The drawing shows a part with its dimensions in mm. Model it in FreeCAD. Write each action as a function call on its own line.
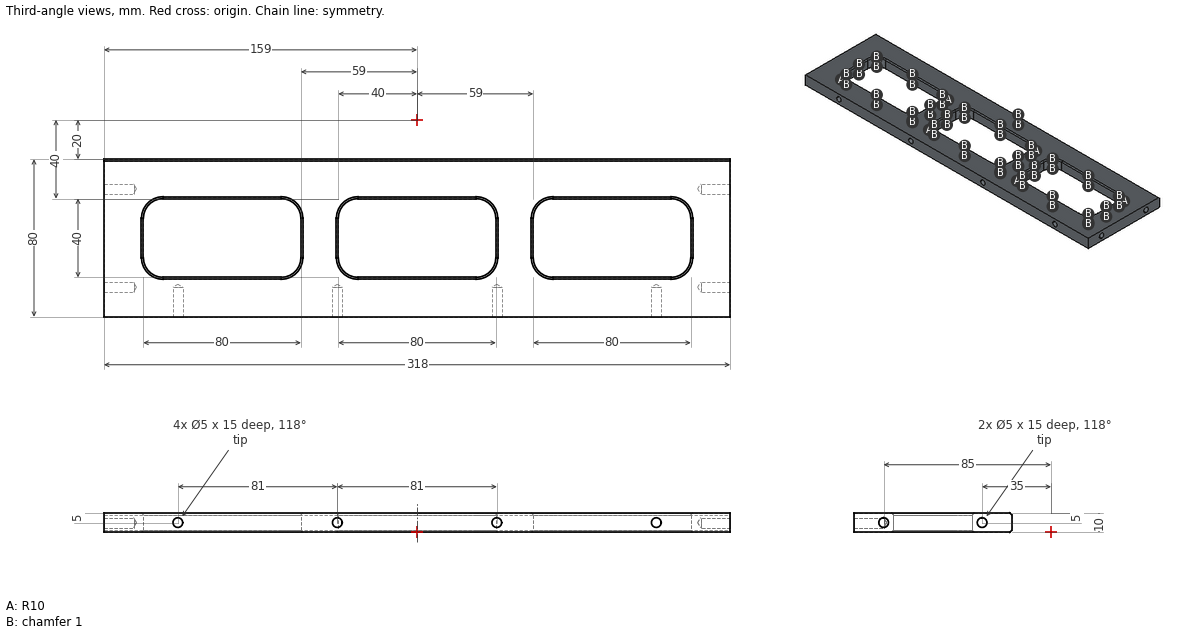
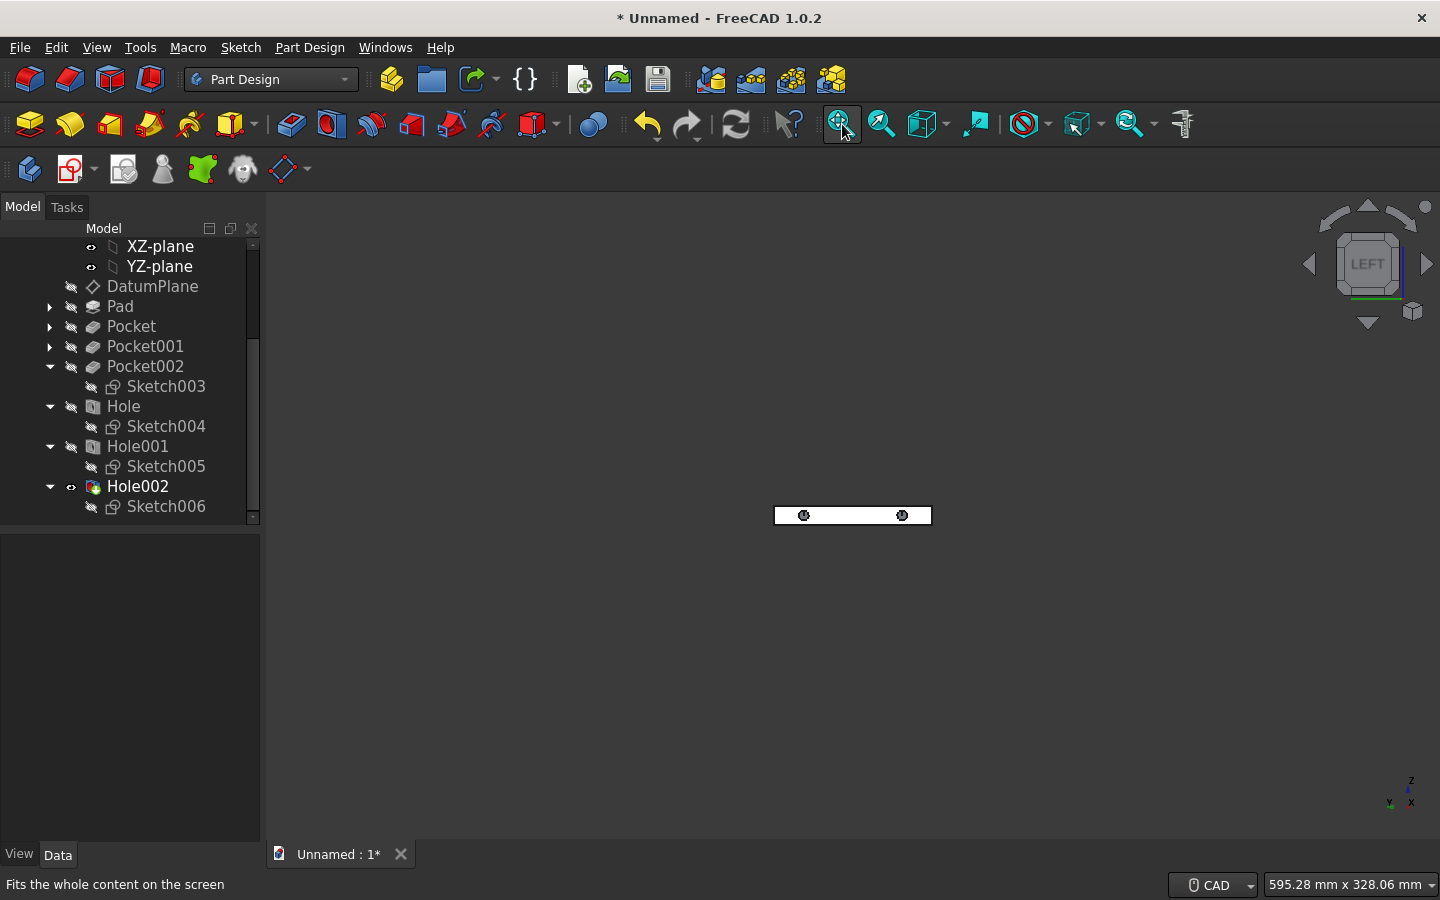
scroll(892, 514, up, 4)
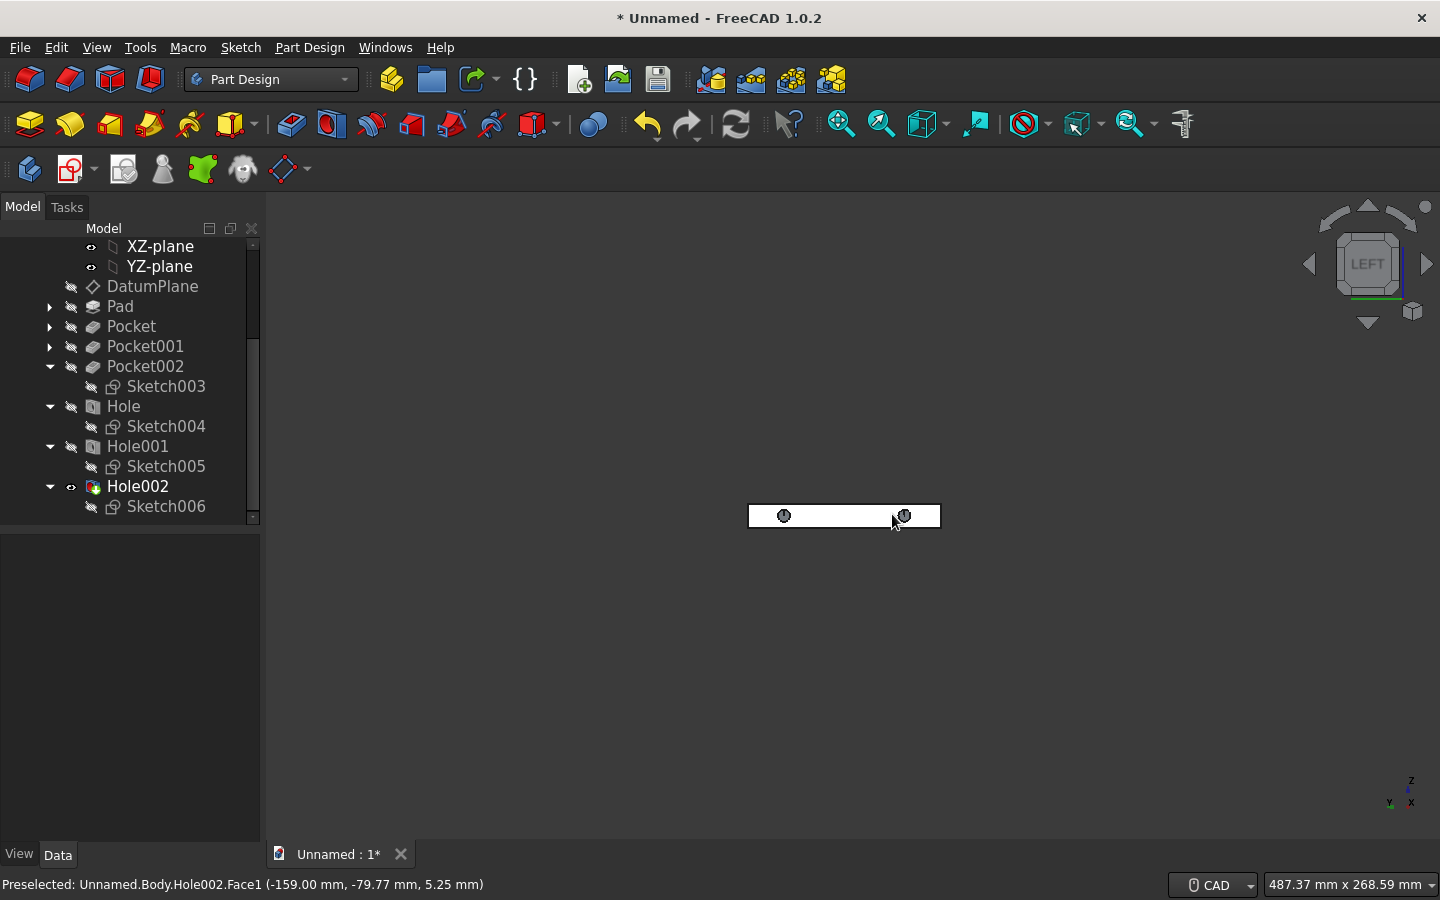
click(842, 124)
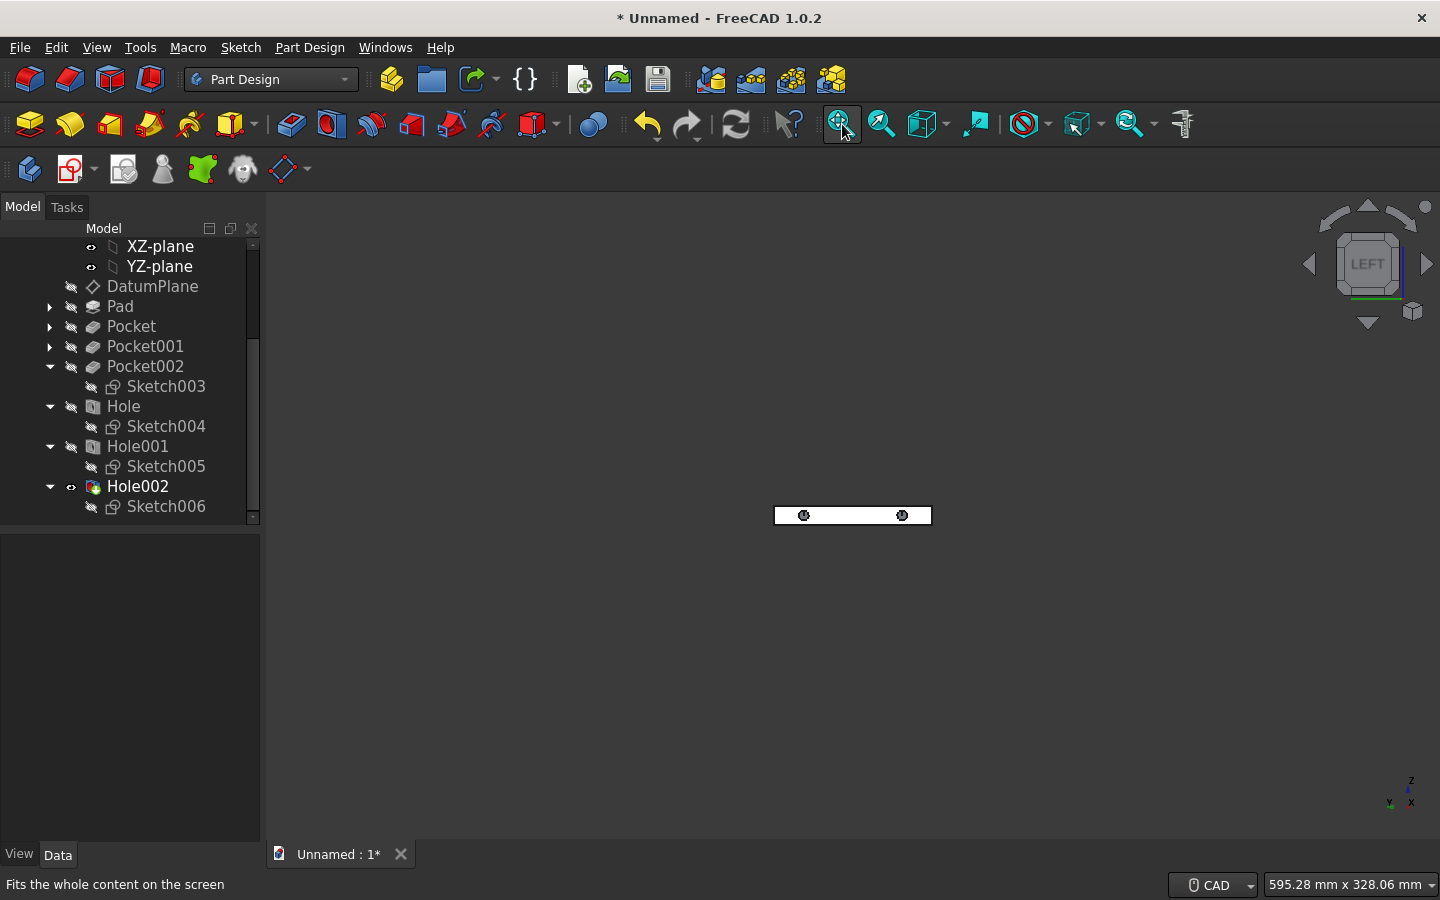
key(v)
key(3)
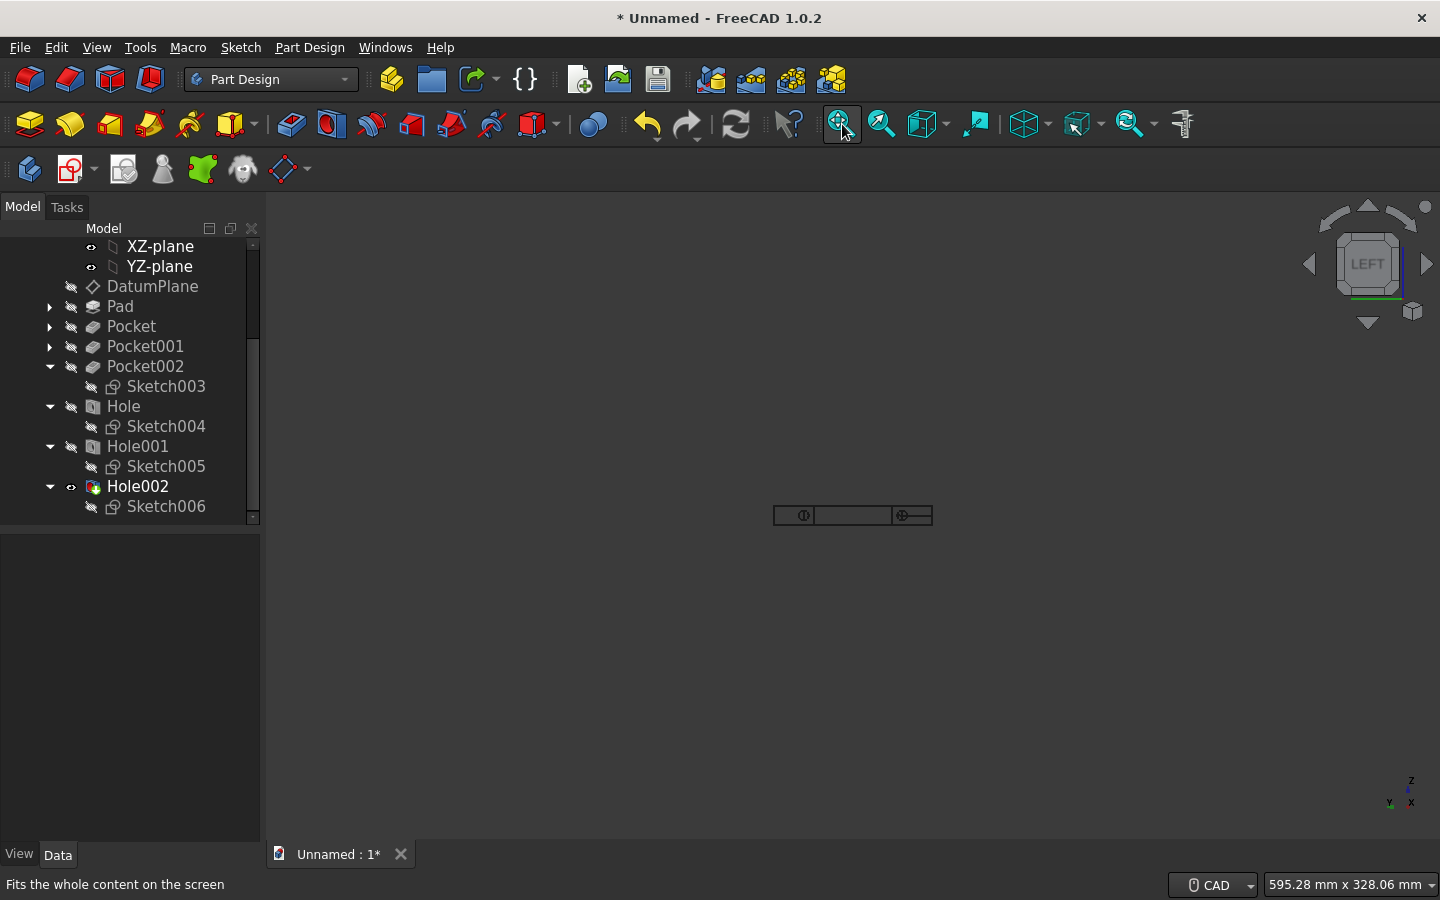
key(0)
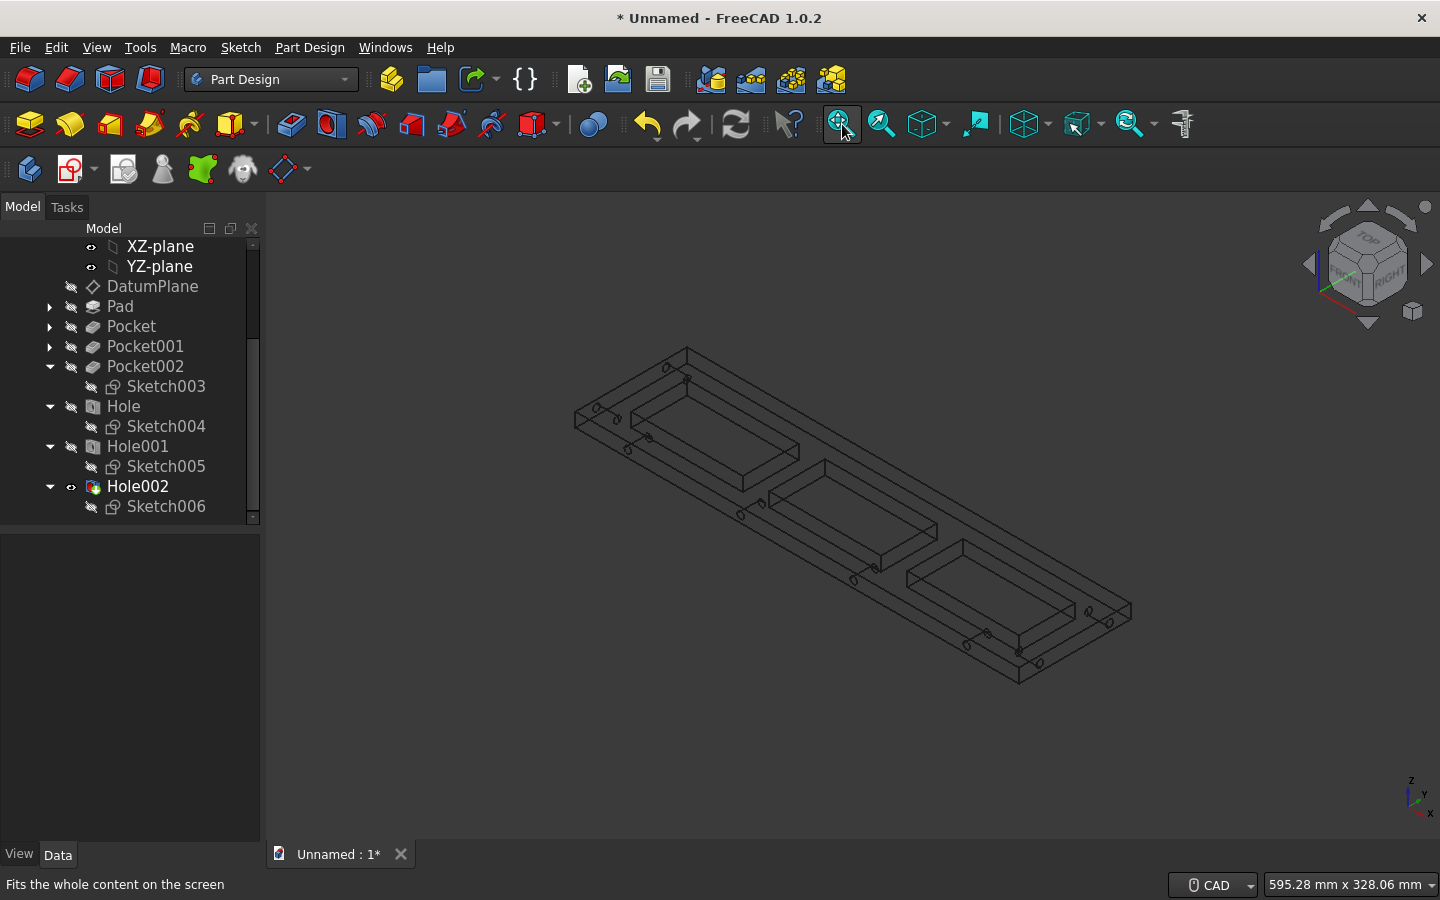
click(825, 466)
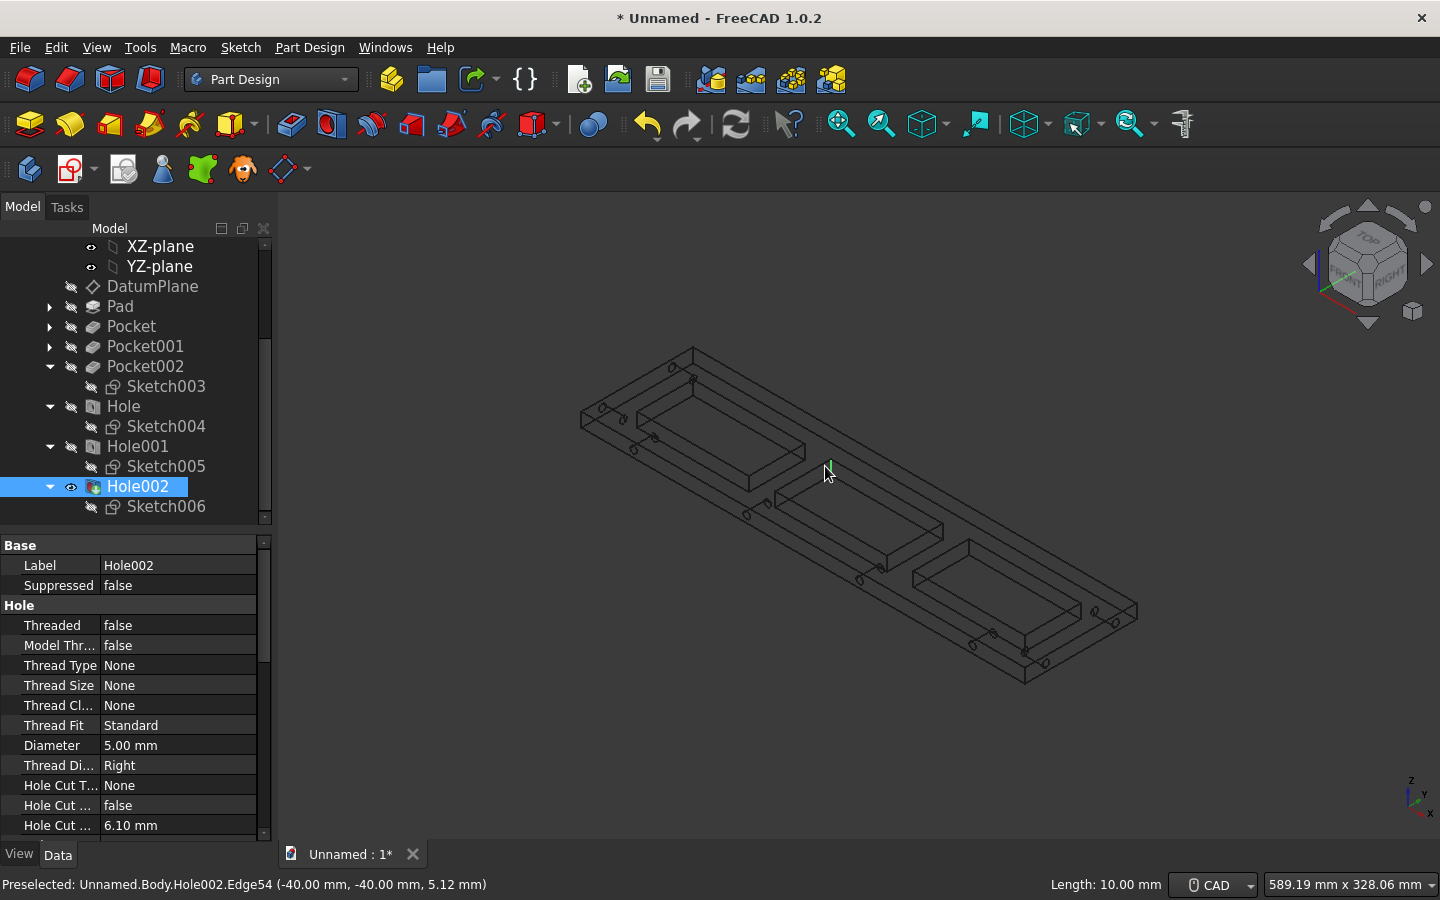
click(943, 531, ctrl)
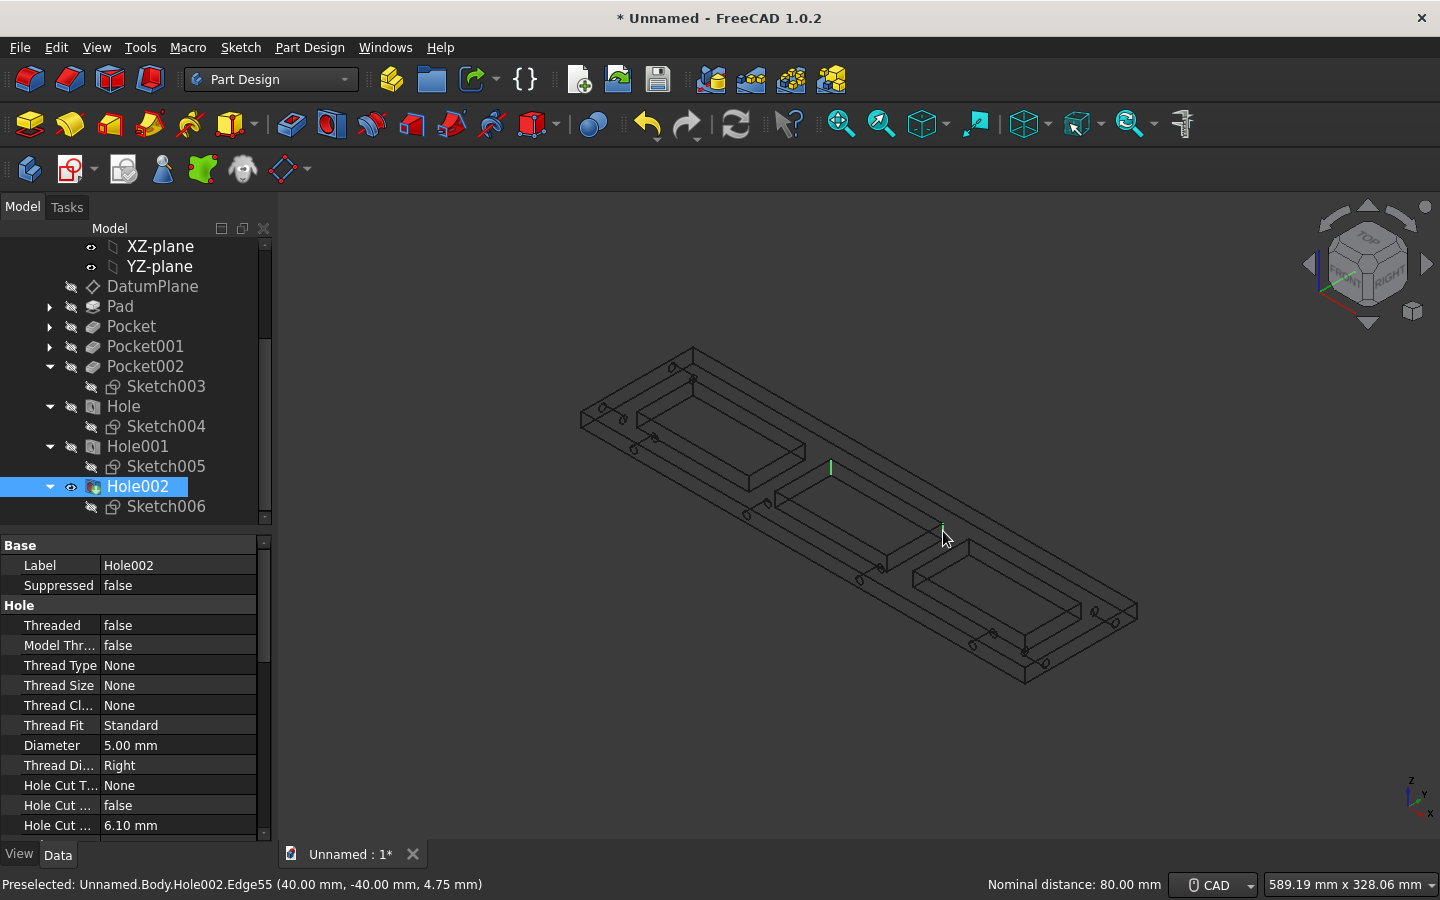
click(913, 578, ctrl)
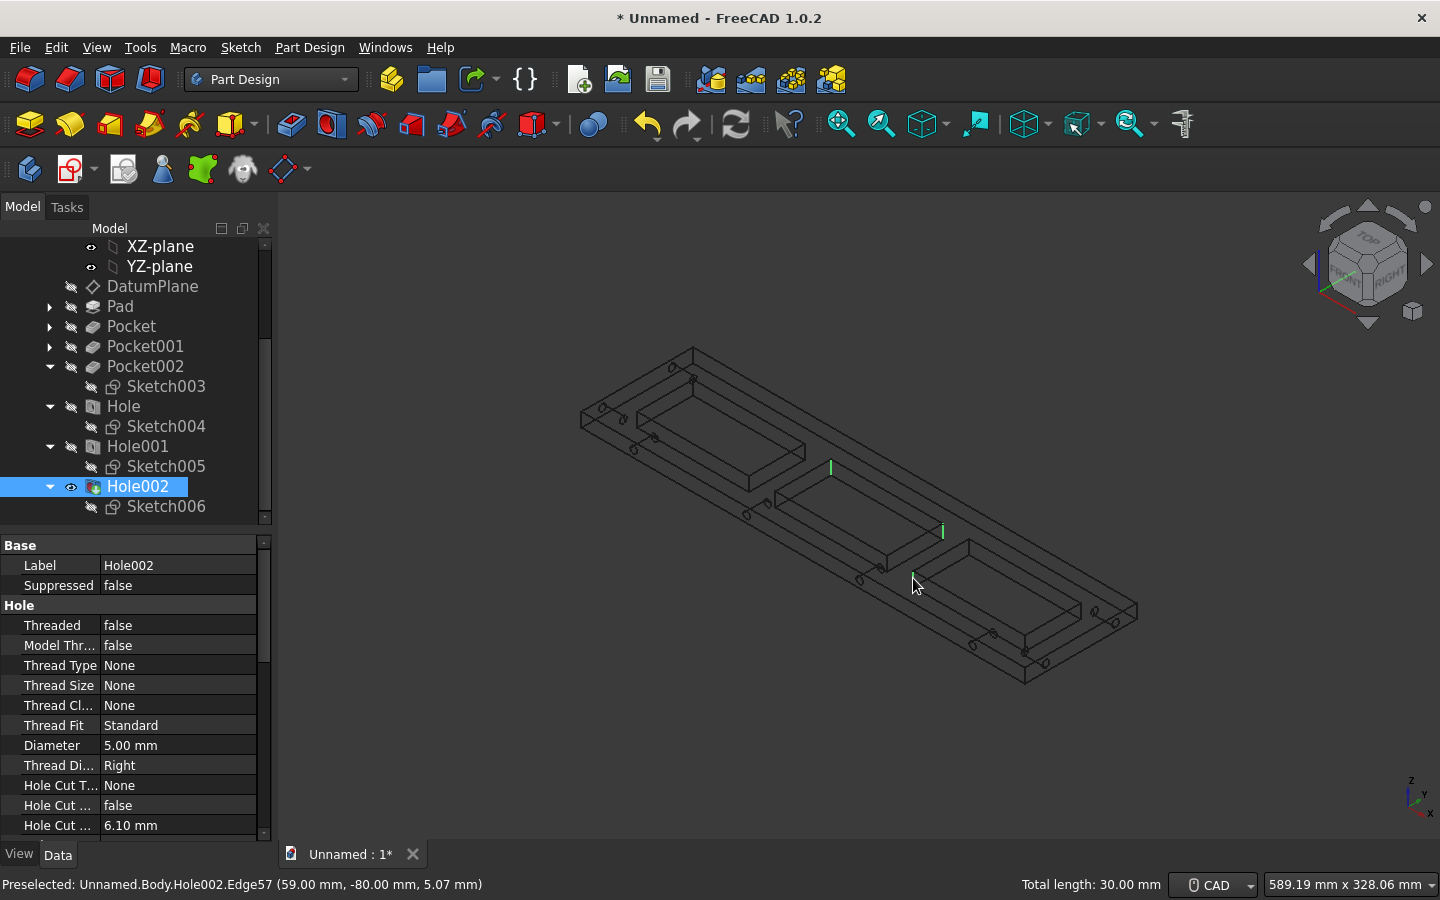
click(969, 546, ctrl)